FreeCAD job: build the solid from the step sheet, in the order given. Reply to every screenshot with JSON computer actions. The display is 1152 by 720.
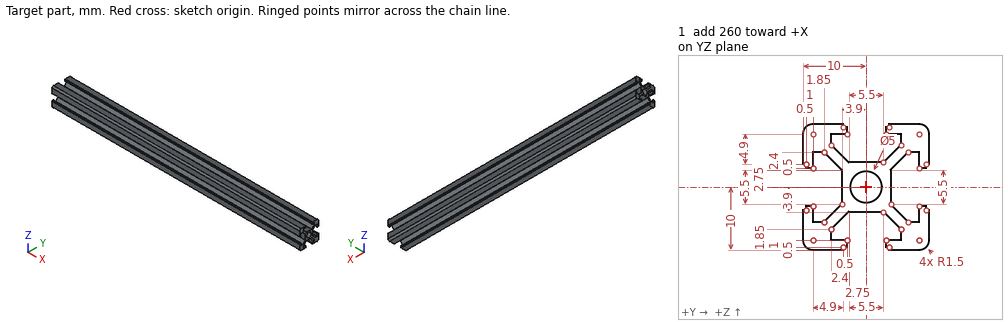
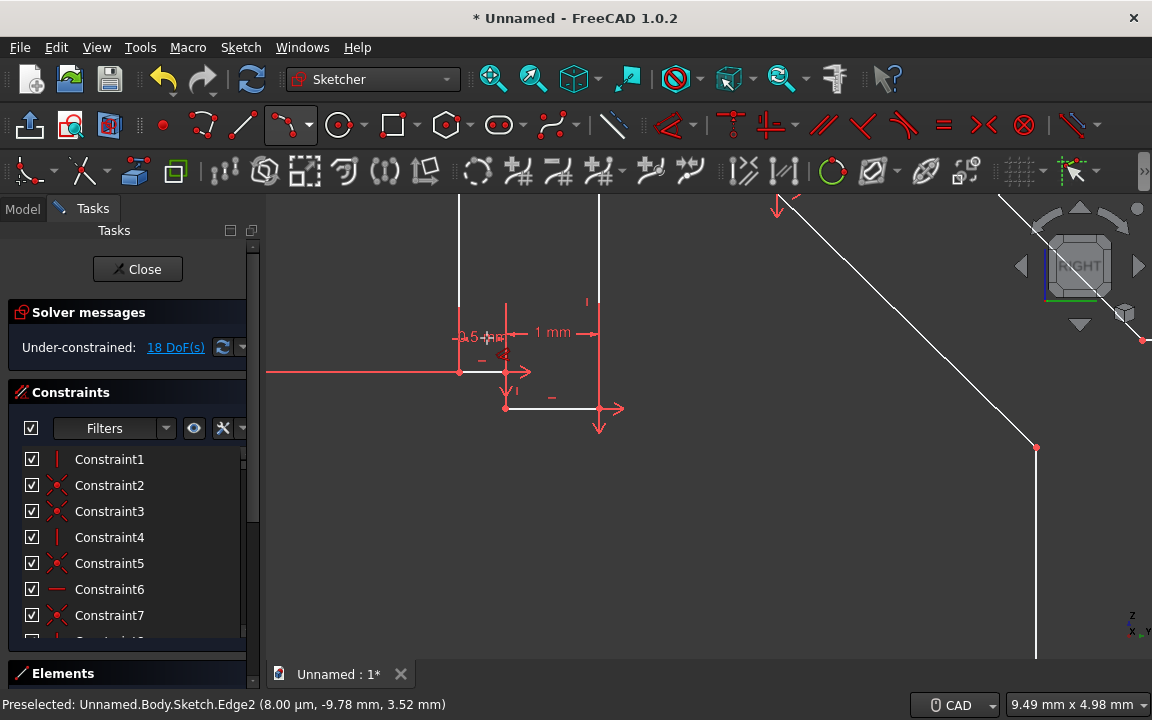
{"action": "scroll", "coordinate": [506, 383], "scroll_direction": "up", "scroll_amount": 2}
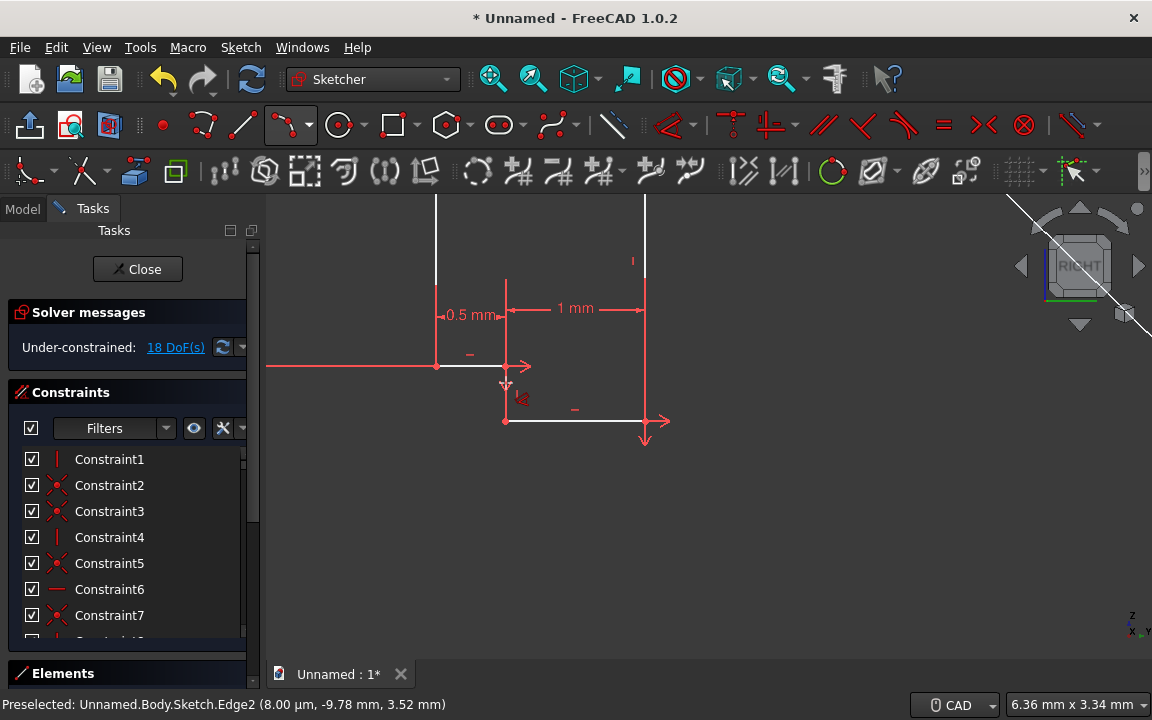
{"action": "left_click", "coordinate": [506, 383]}
{"action": "left_click", "coordinate": [472, 394]}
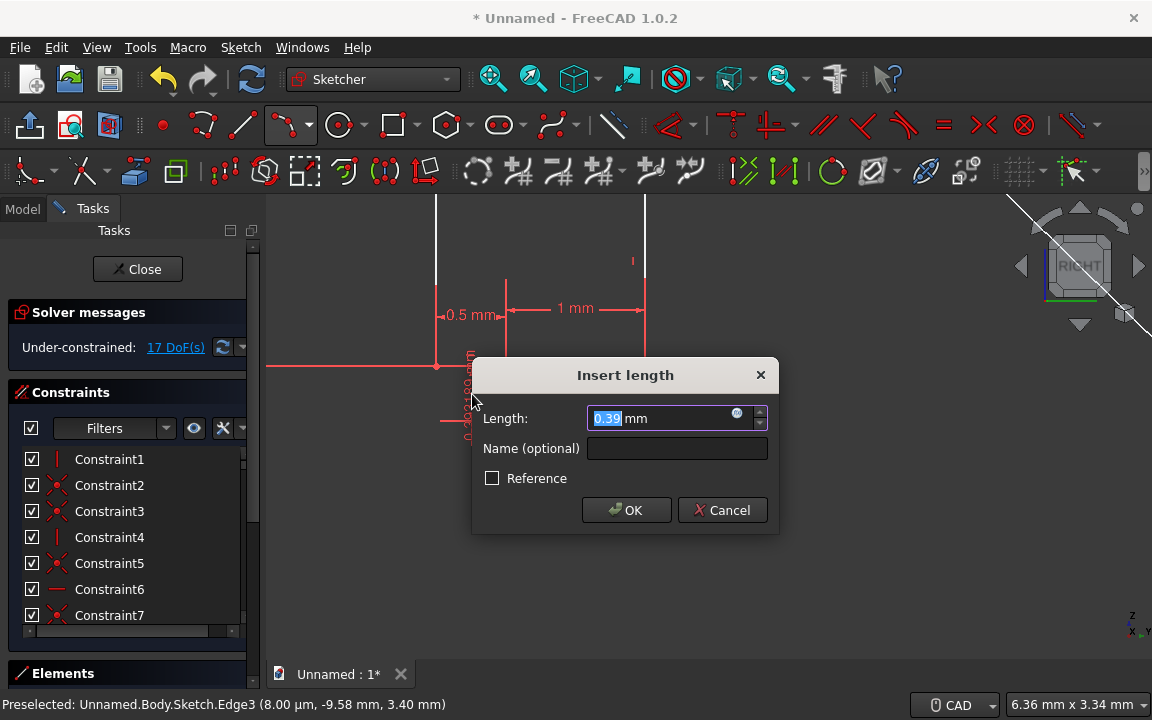
{"action": "type", "text": "0.5"}
{"action": "key", "text": "Return"}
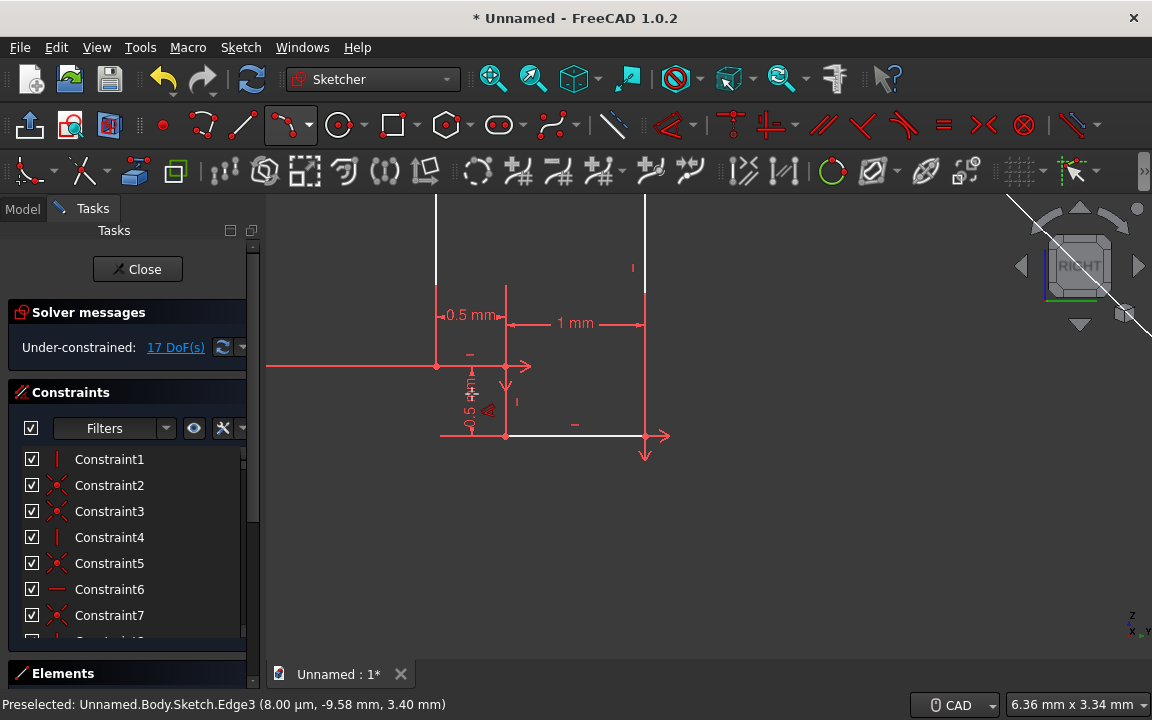
{"action": "scroll", "coordinate": [491, 373], "scroll_direction": "down", "scroll_amount": 11}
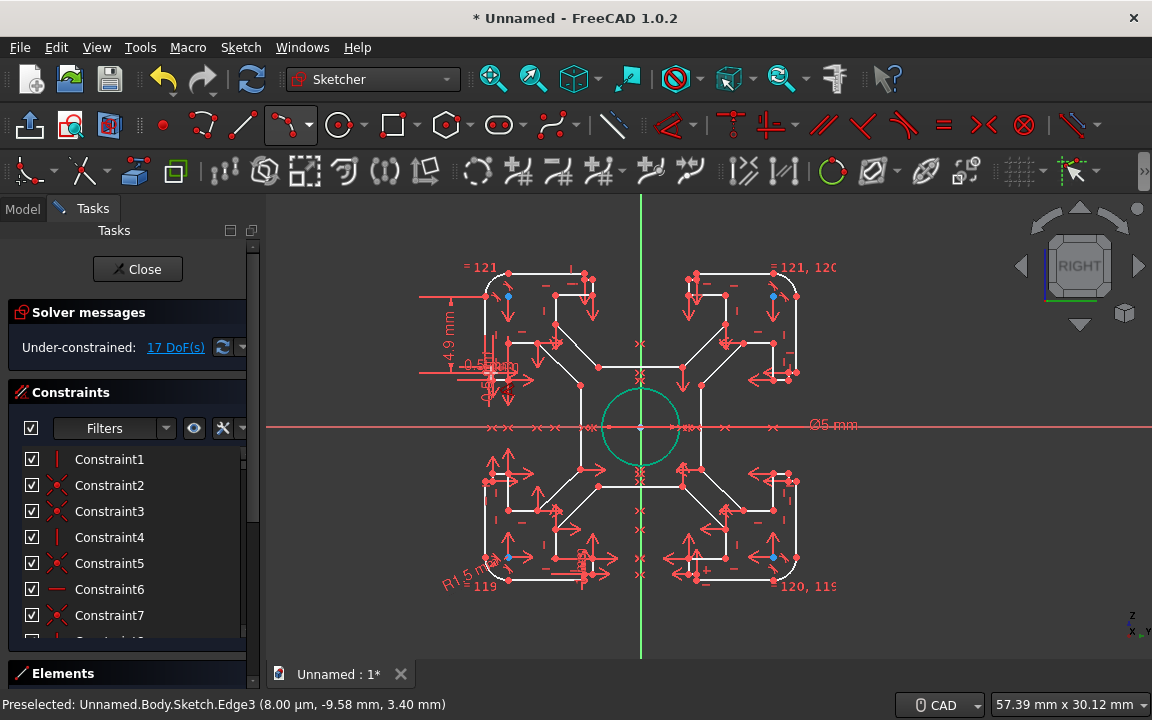
{"action": "scroll", "coordinate": [508, 369], "scroll_direction": "up", "scroll_amount": 2}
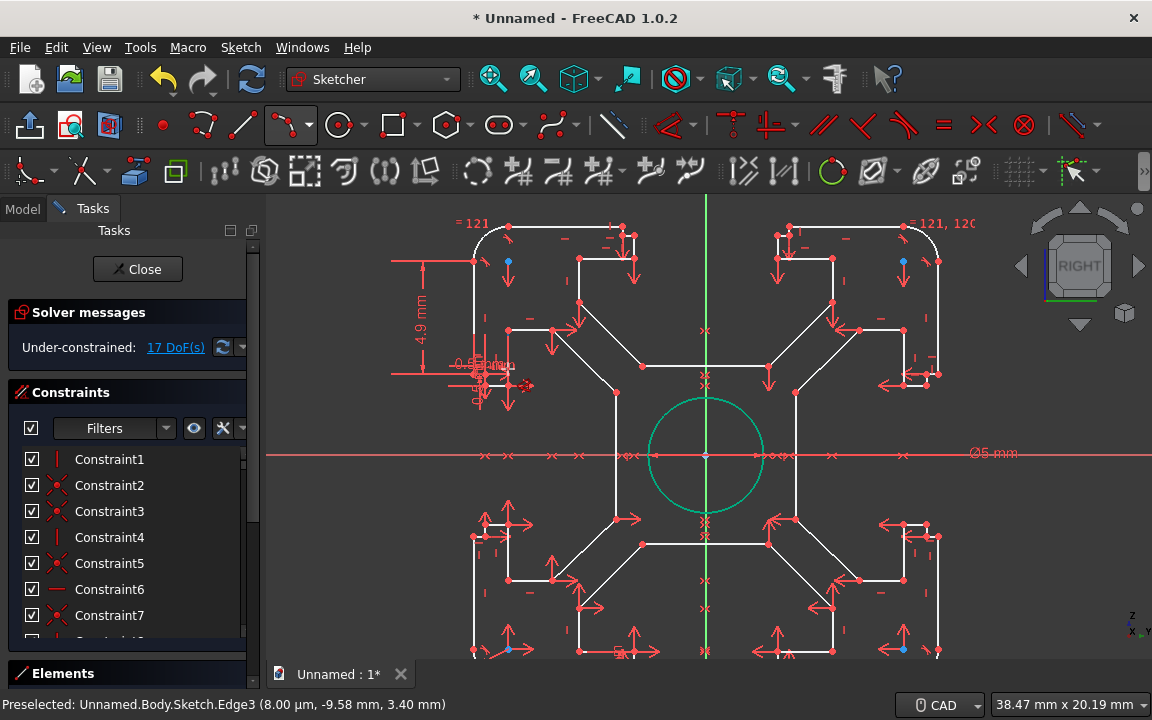
{"action": "left_click", "coordinate": [508, 369]}
{"action": "left_click", "coordinate": [450, 338]}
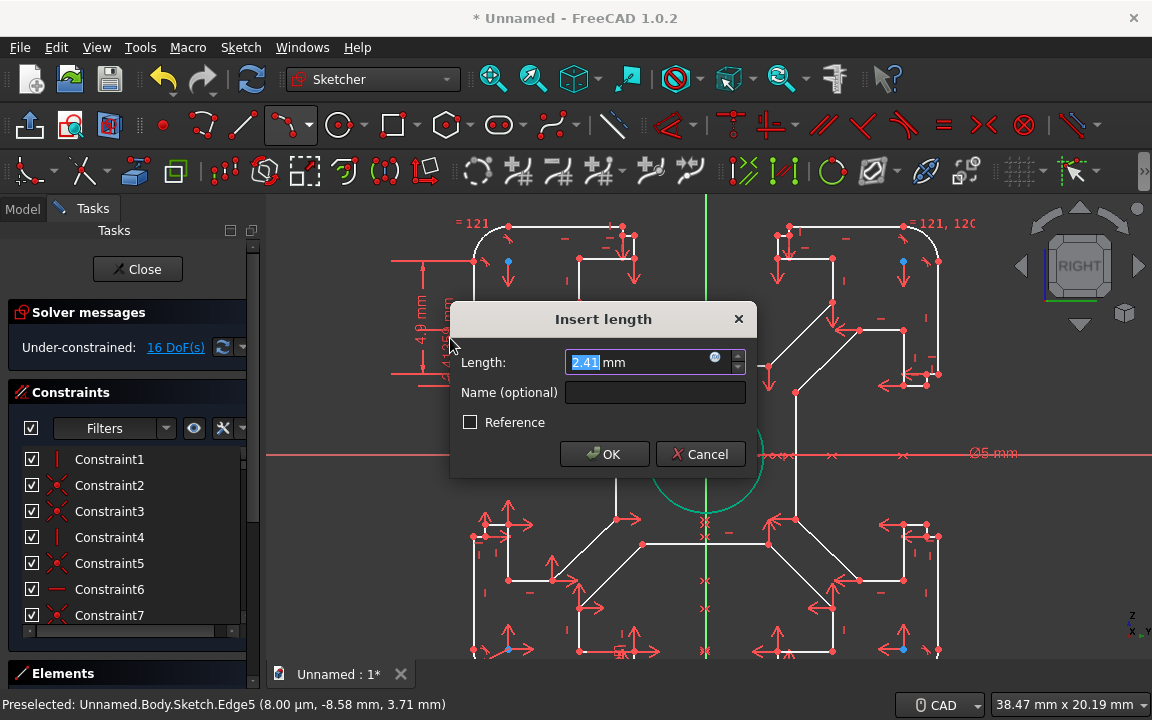
{"action": "type", "text": "2.4"}
{"action": "key", "text": "Return"}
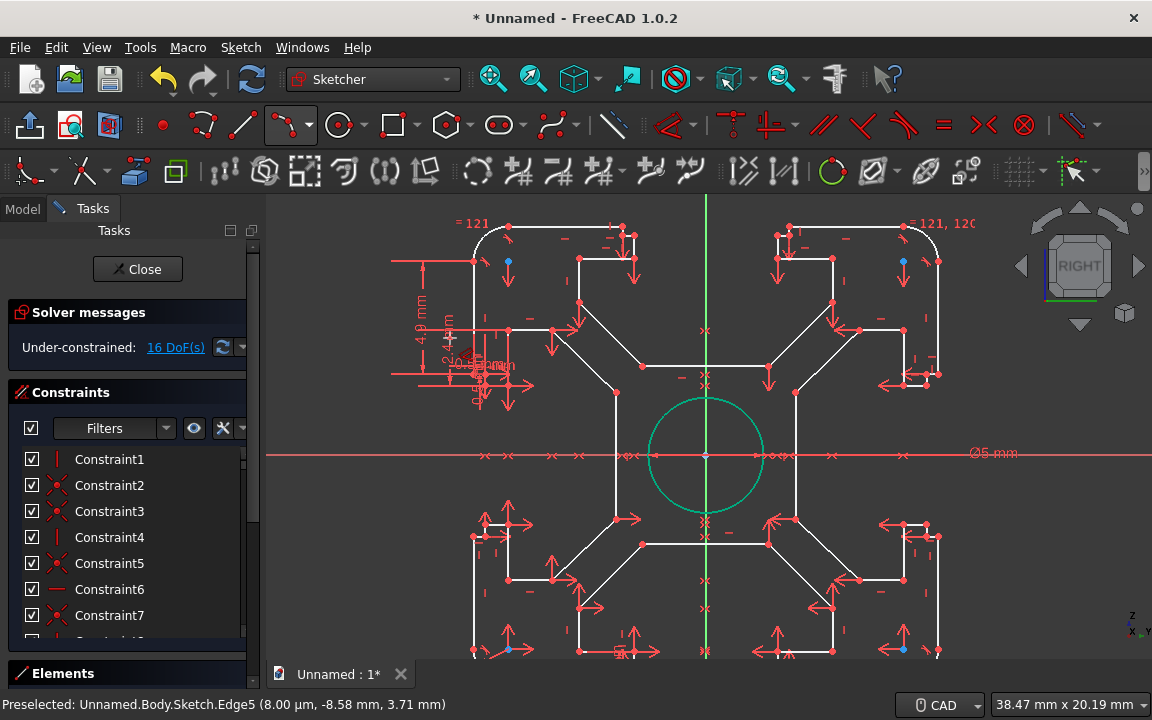
{"action": "left_click", "coordinate": [616, 431]}
{"action": "left_click", "coordinate": [582, 427]}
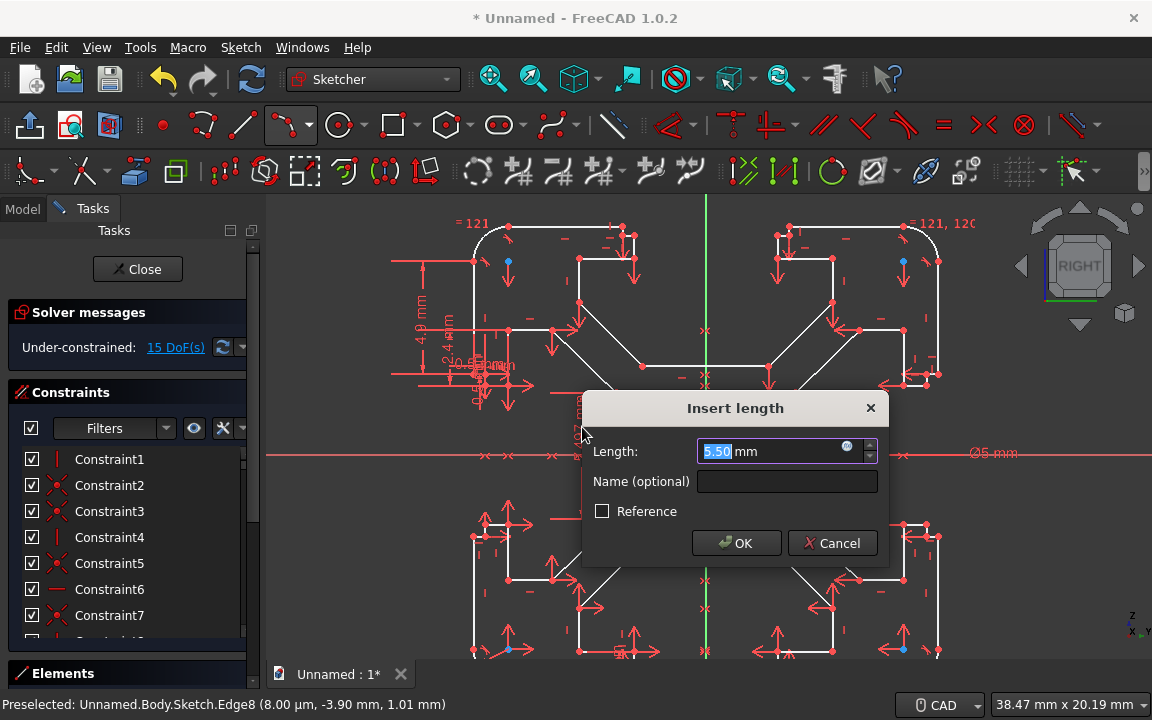
{"action": "type", "text": "5.5"}
{"action": "key", "text": "Return"}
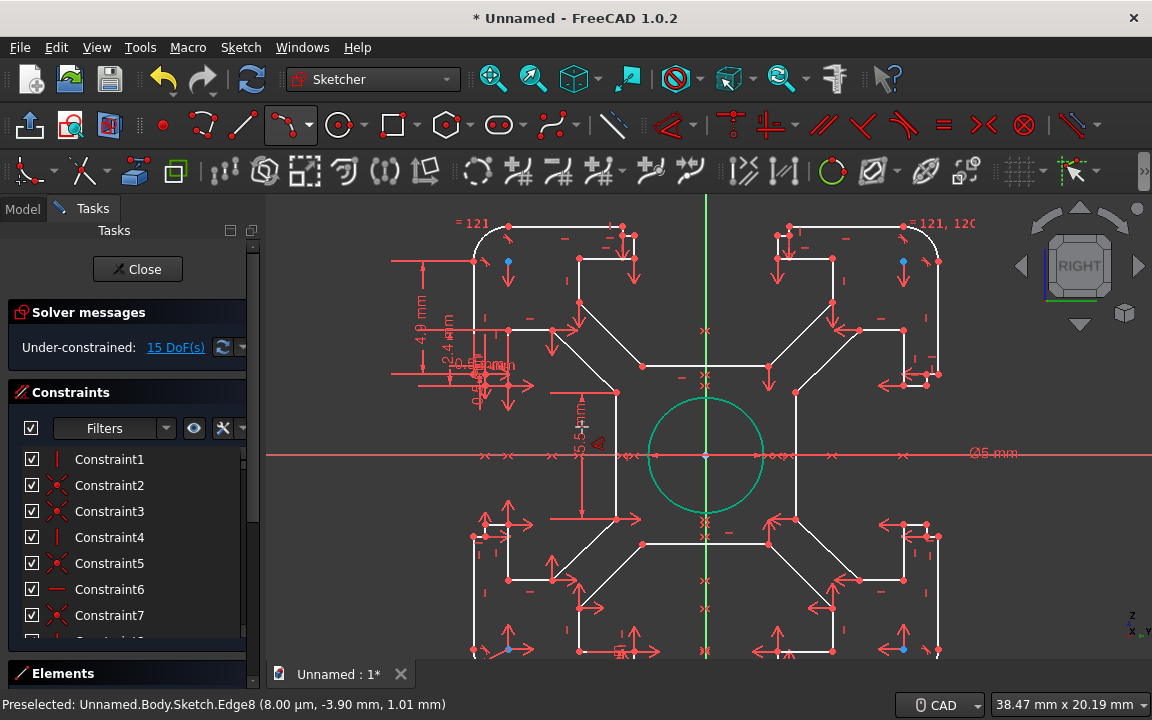
{"action": "scroll", "coordinate": [507, 368], "scroll_direction": "down", "scroll_amount": 2}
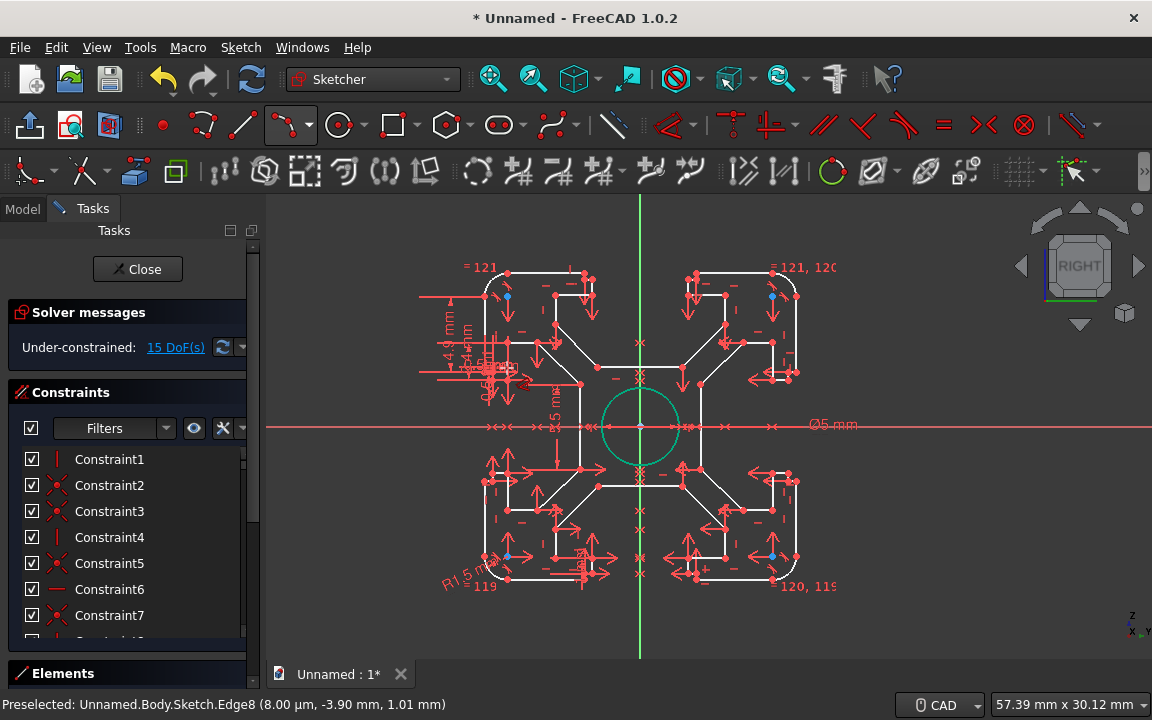
{"action": "left_click", "coordinate": [531, 580]}
{"action": "left_click", "coordinate": [546, 614]}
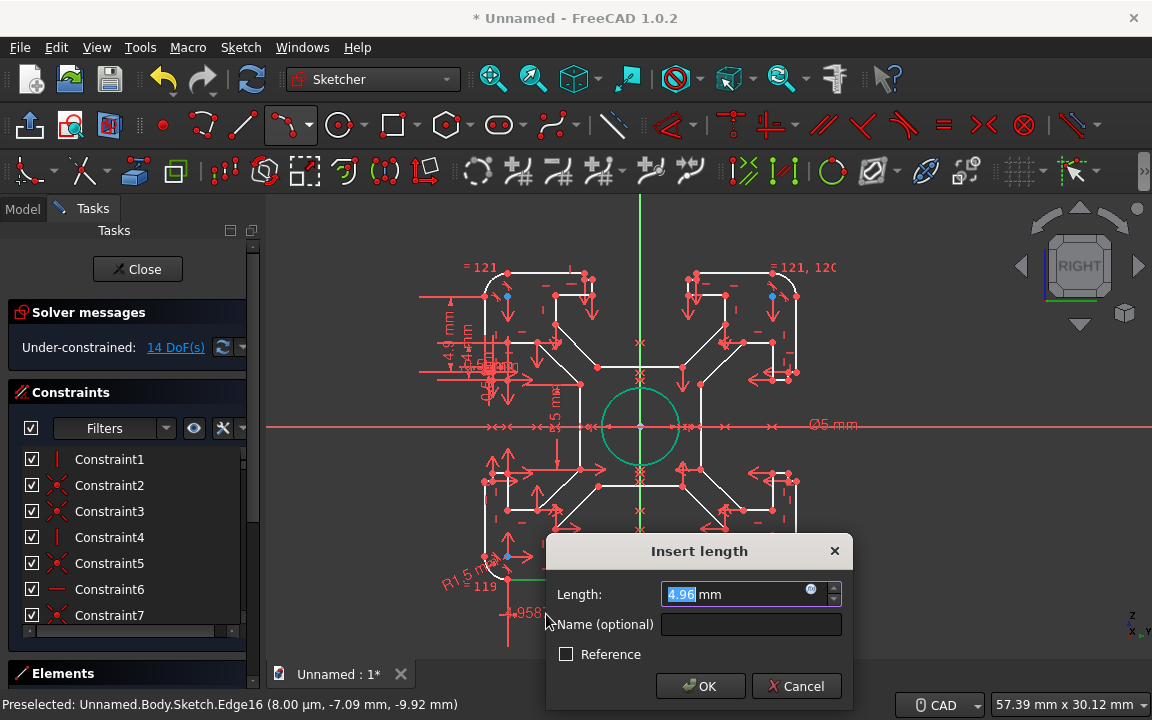
{"action": "type", "text": "4.9"}
{"action": "key", "text": "Return"}